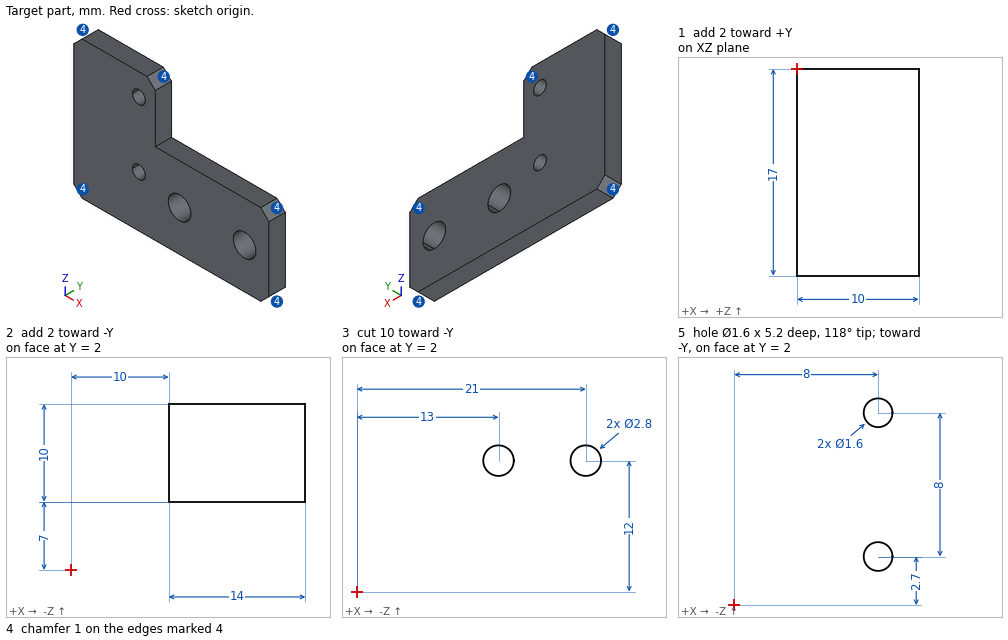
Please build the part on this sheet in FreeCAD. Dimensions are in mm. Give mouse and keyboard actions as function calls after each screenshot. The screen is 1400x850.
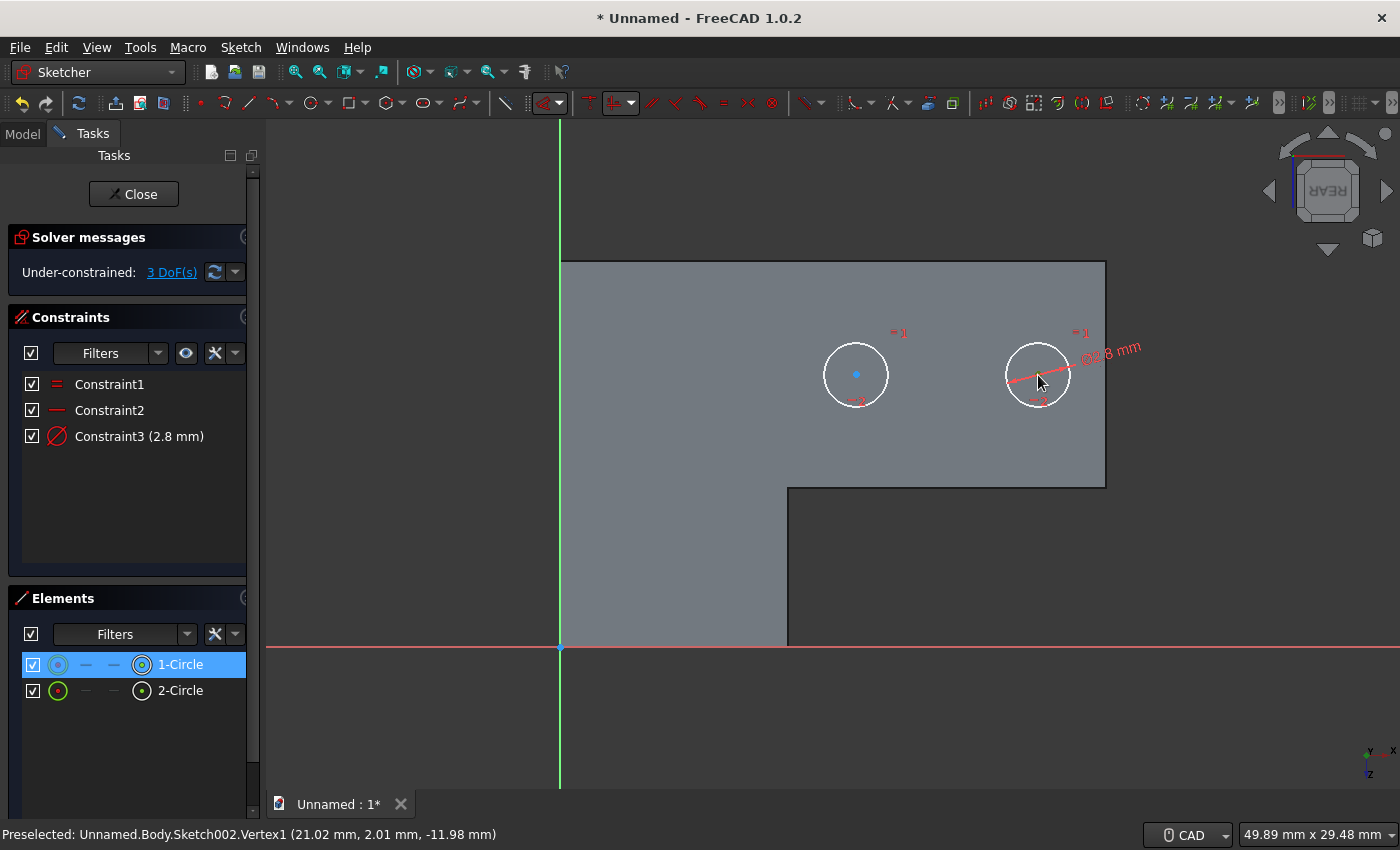
click(562, 104)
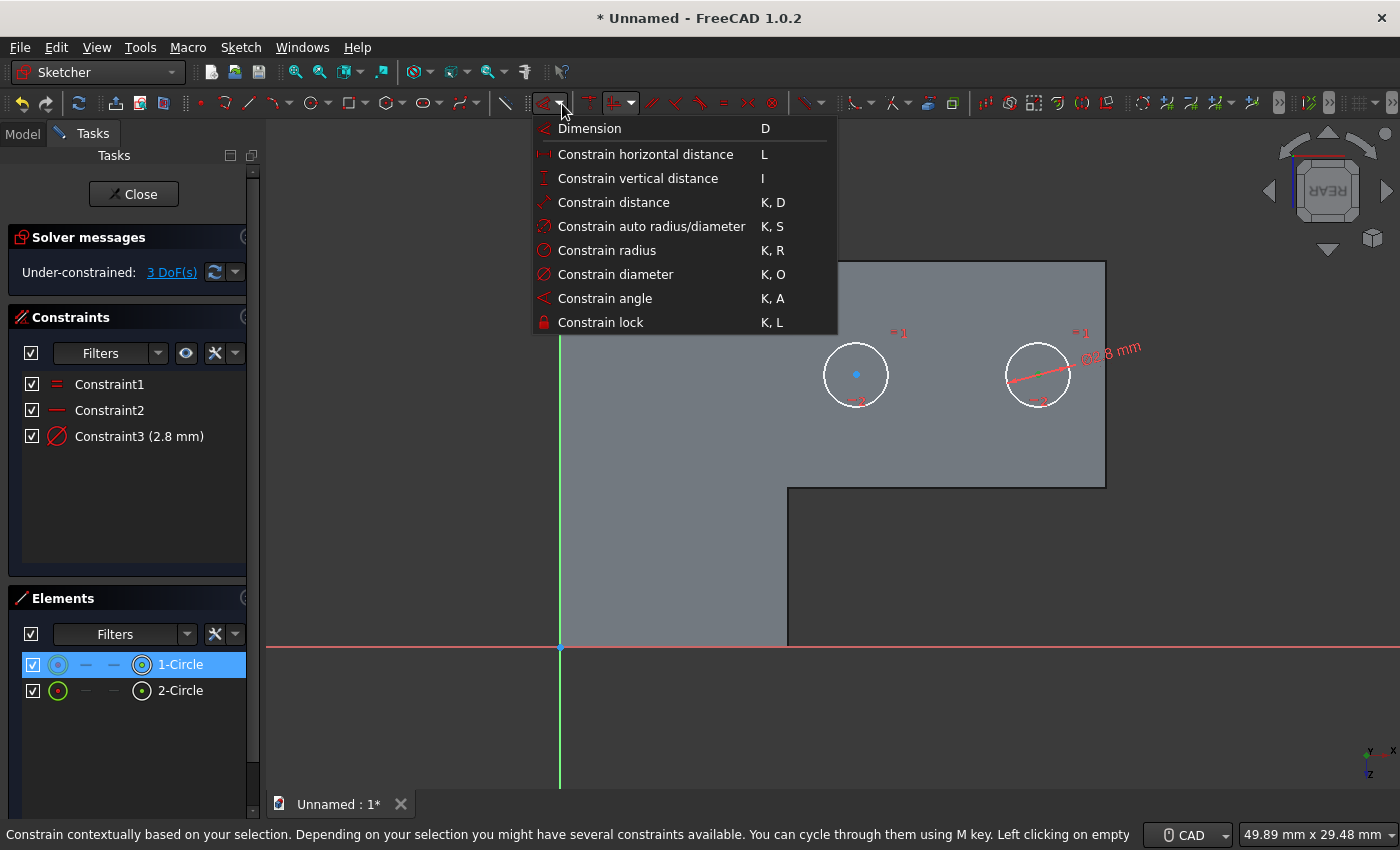
click(685, 154)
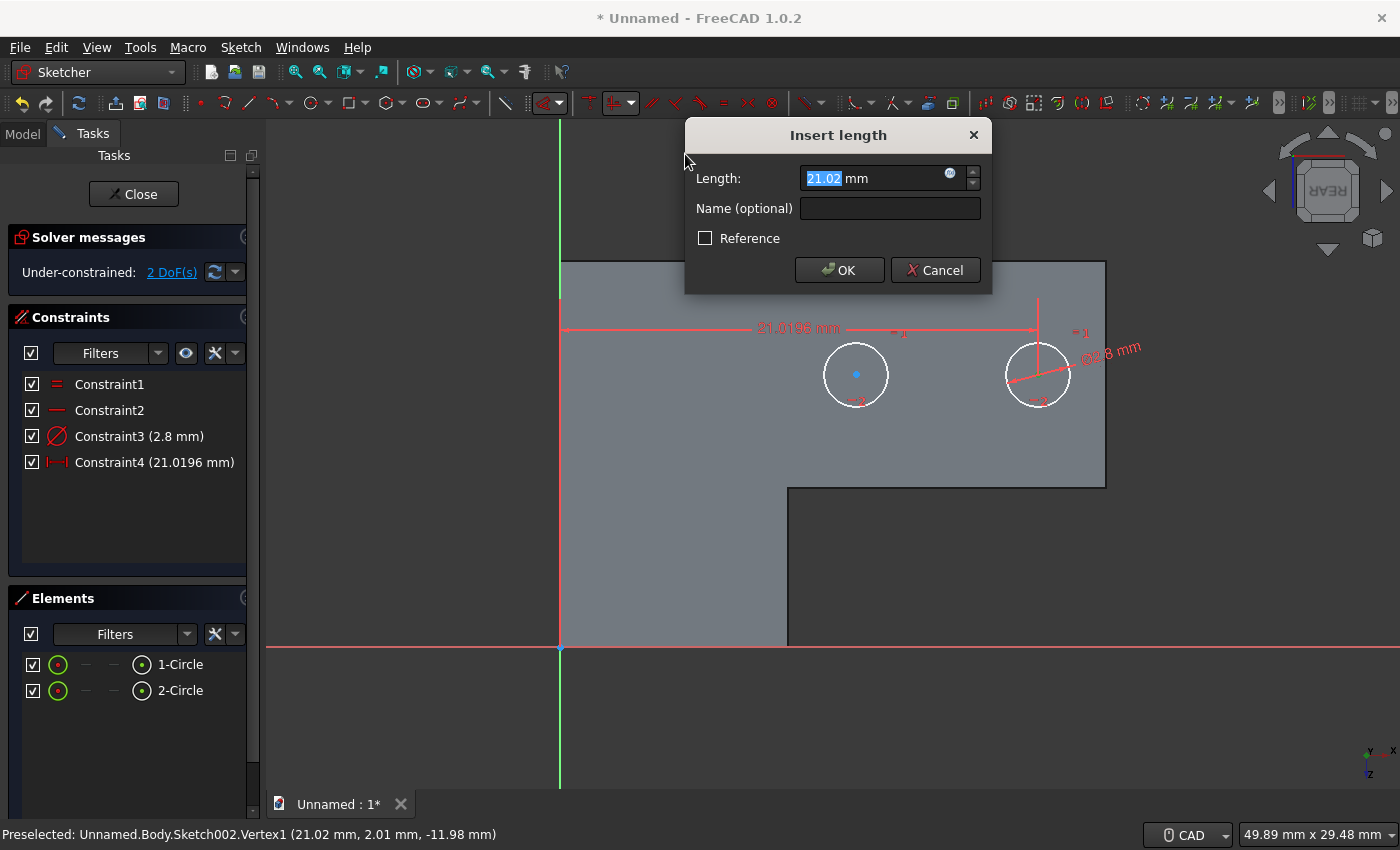
text(21)
key(Return)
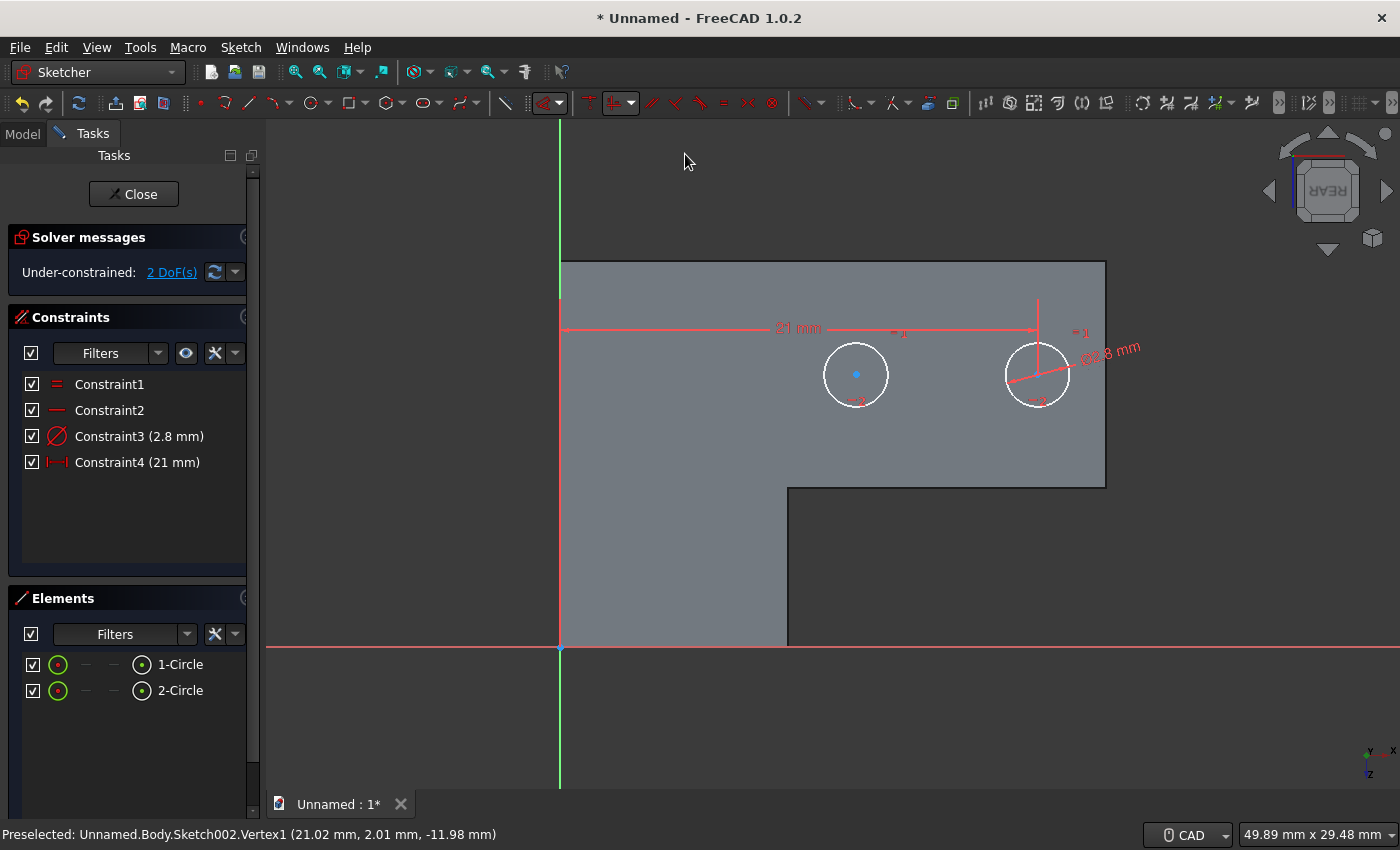
click(1038, 375)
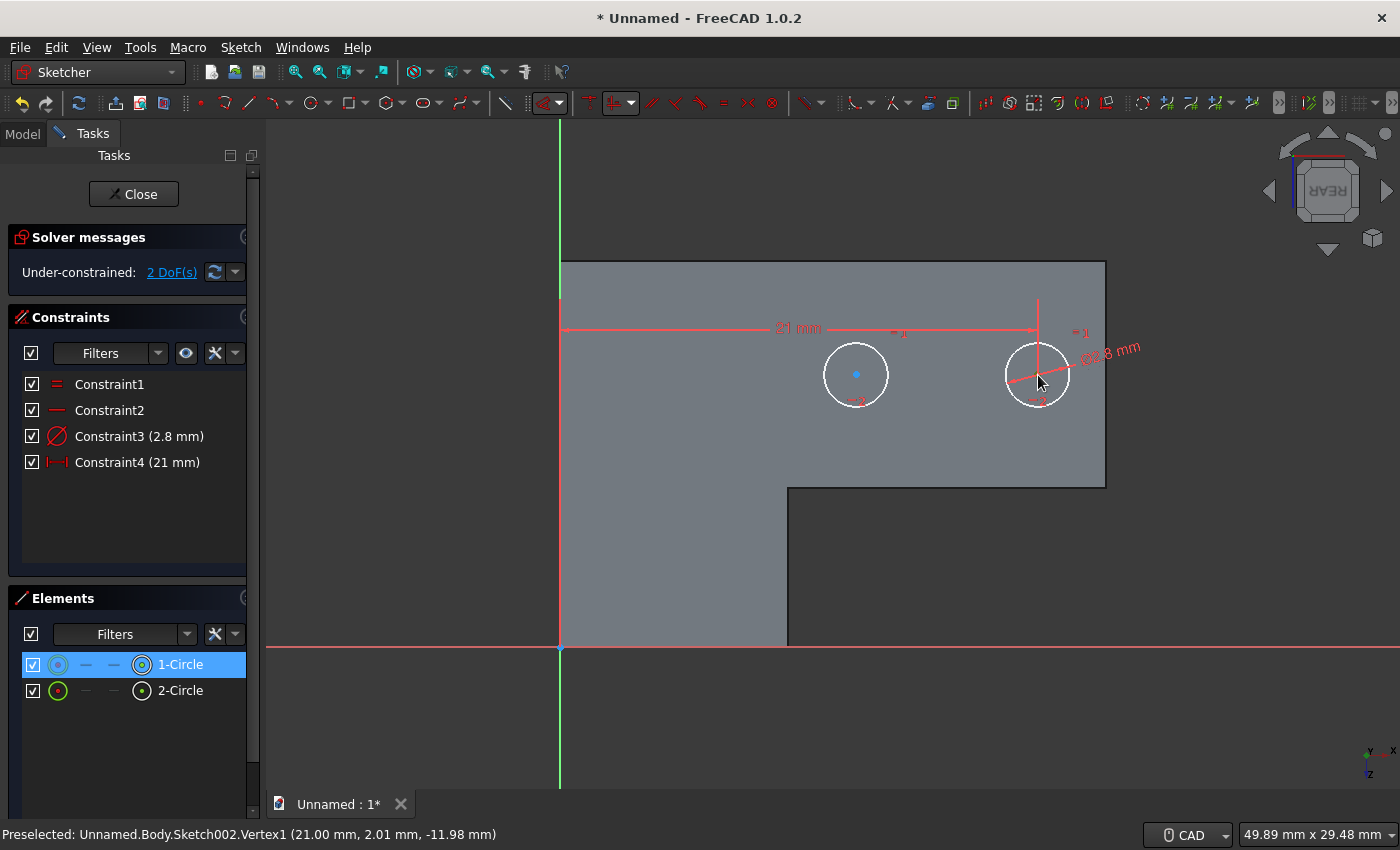
click(562, 104)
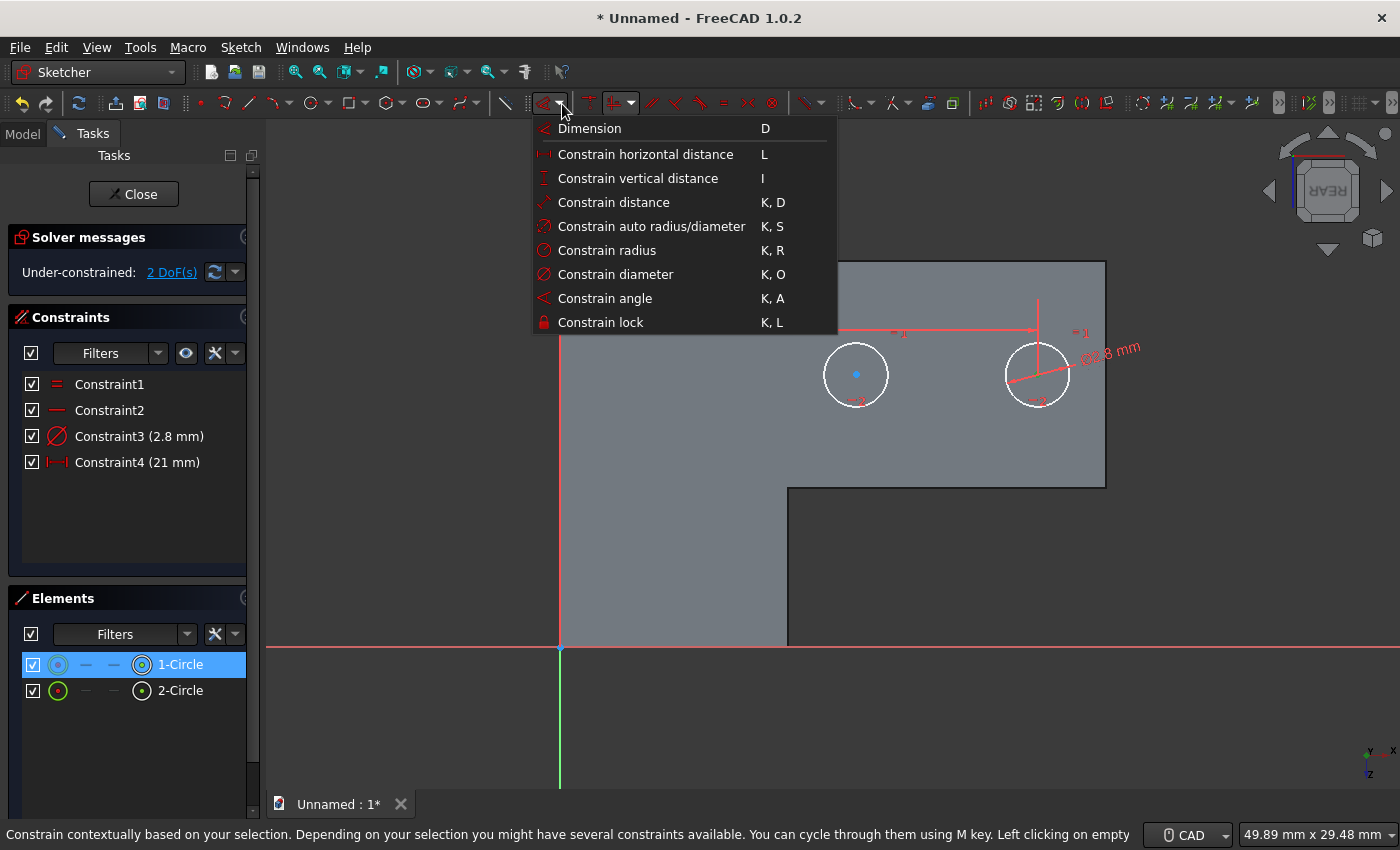
click(685, 178)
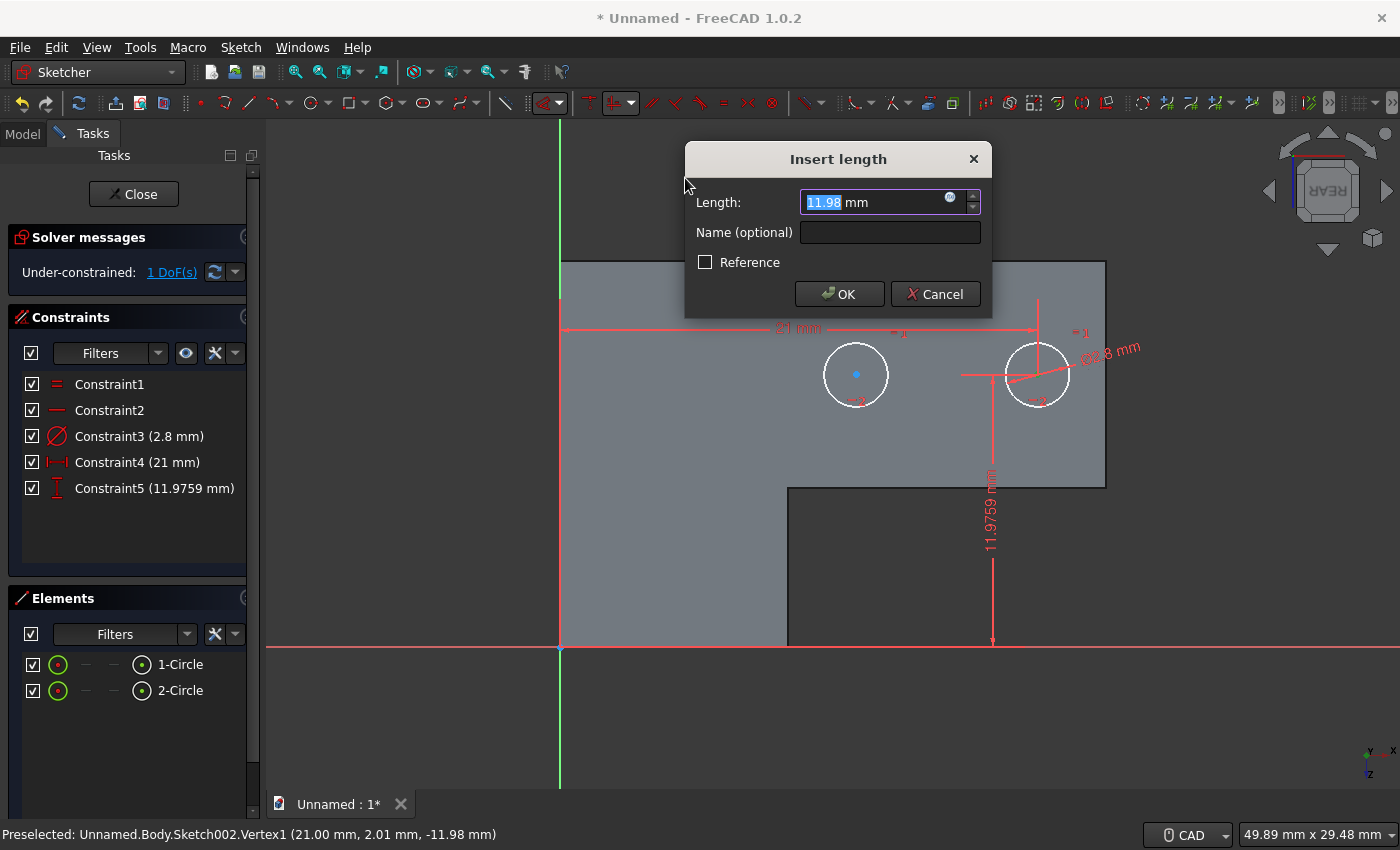
text(12)
key(Return)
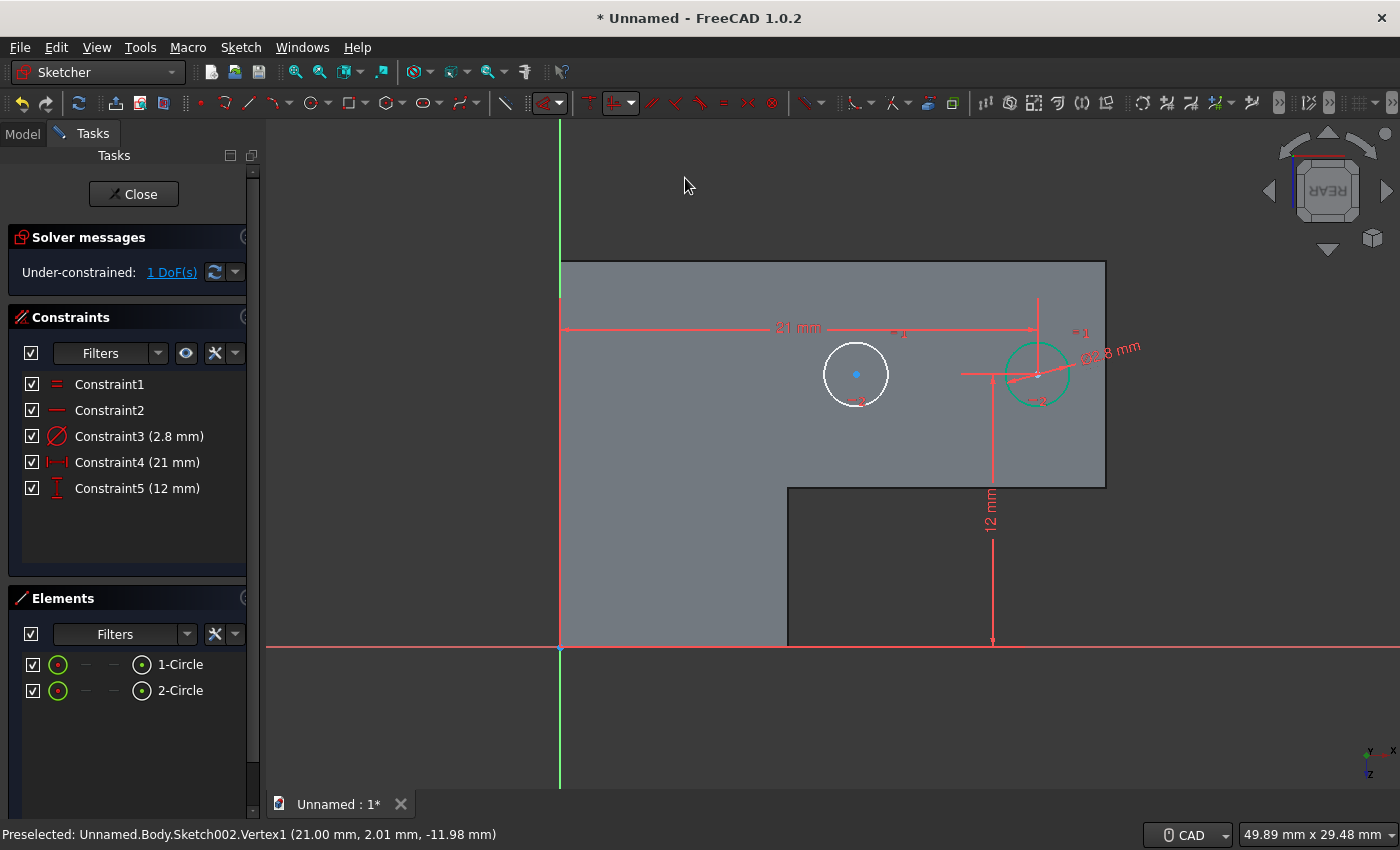
click(856, 374)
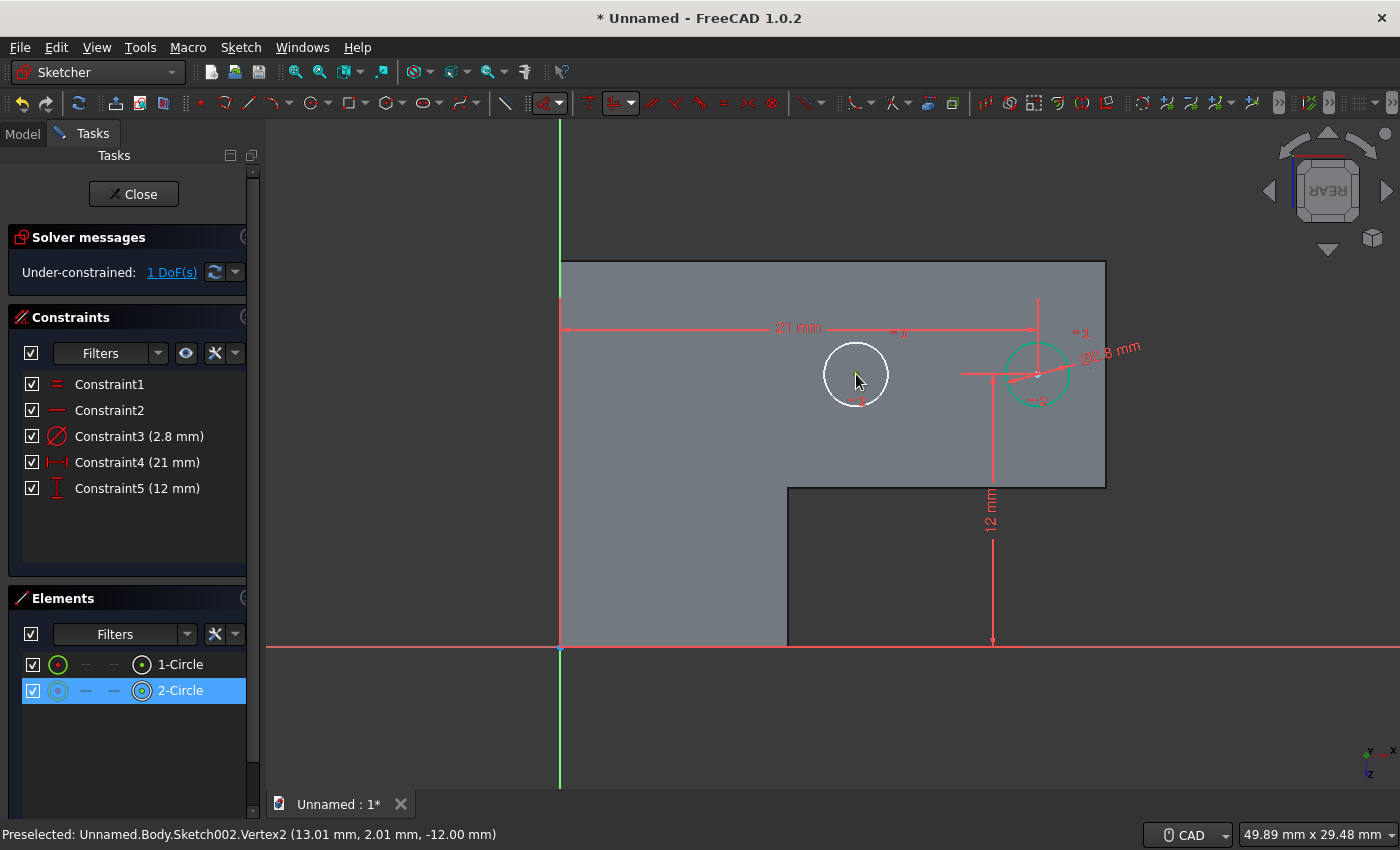
key(l)